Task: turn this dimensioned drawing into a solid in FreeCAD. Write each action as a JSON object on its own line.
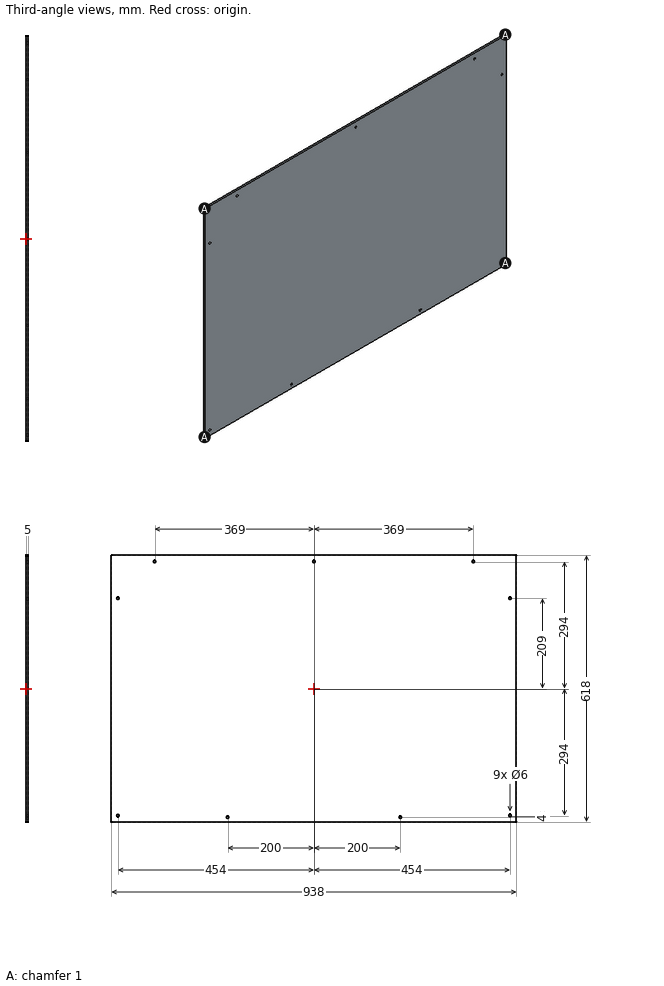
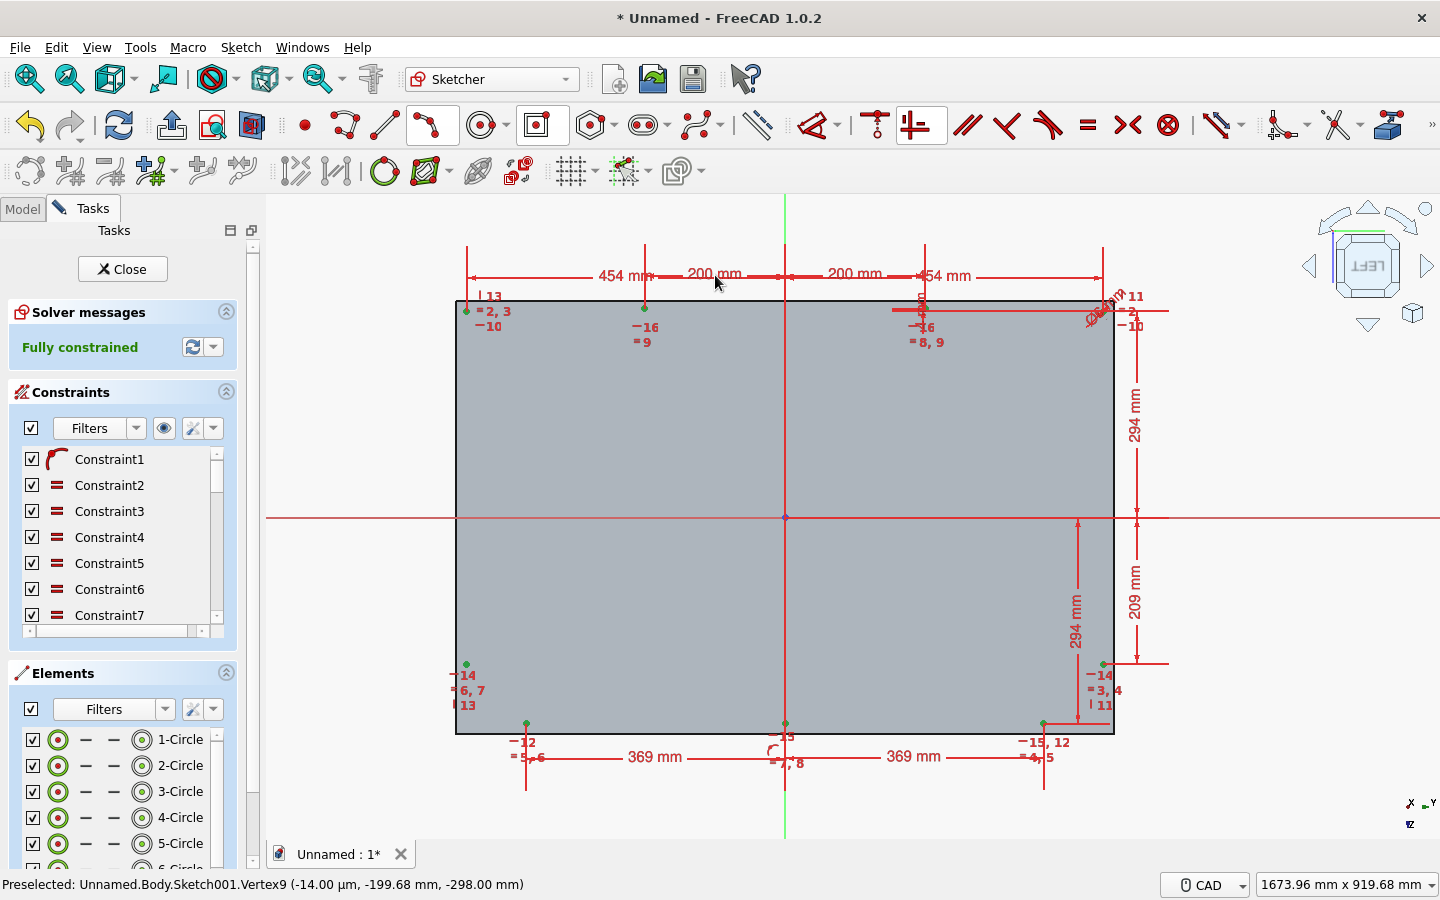
{"action": "left_click", "coordinate": [123, 269]}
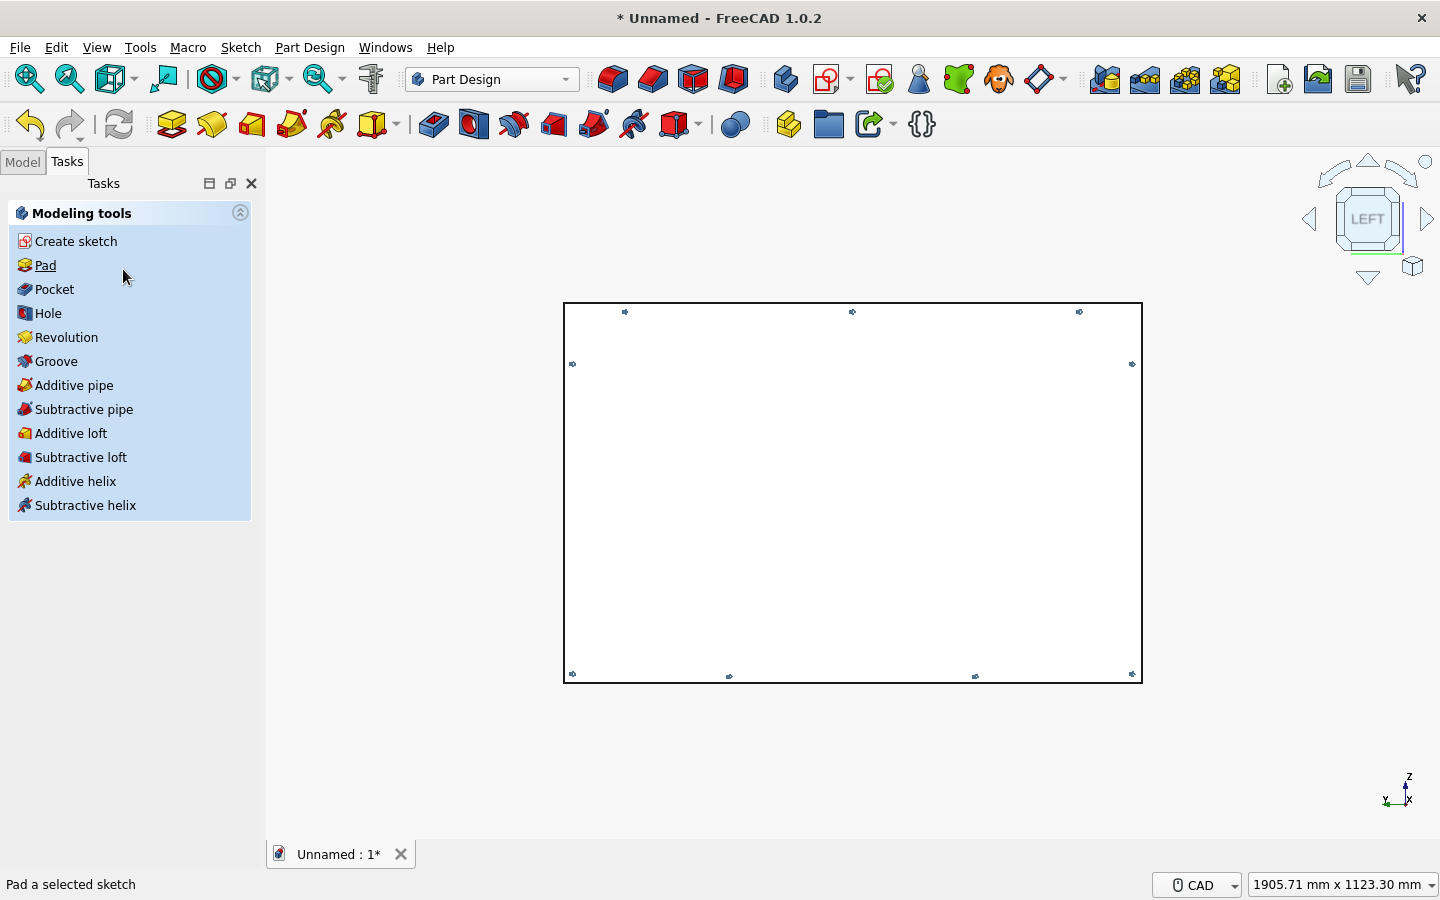
{"action": "left_click", "coordinate": [434, 124]}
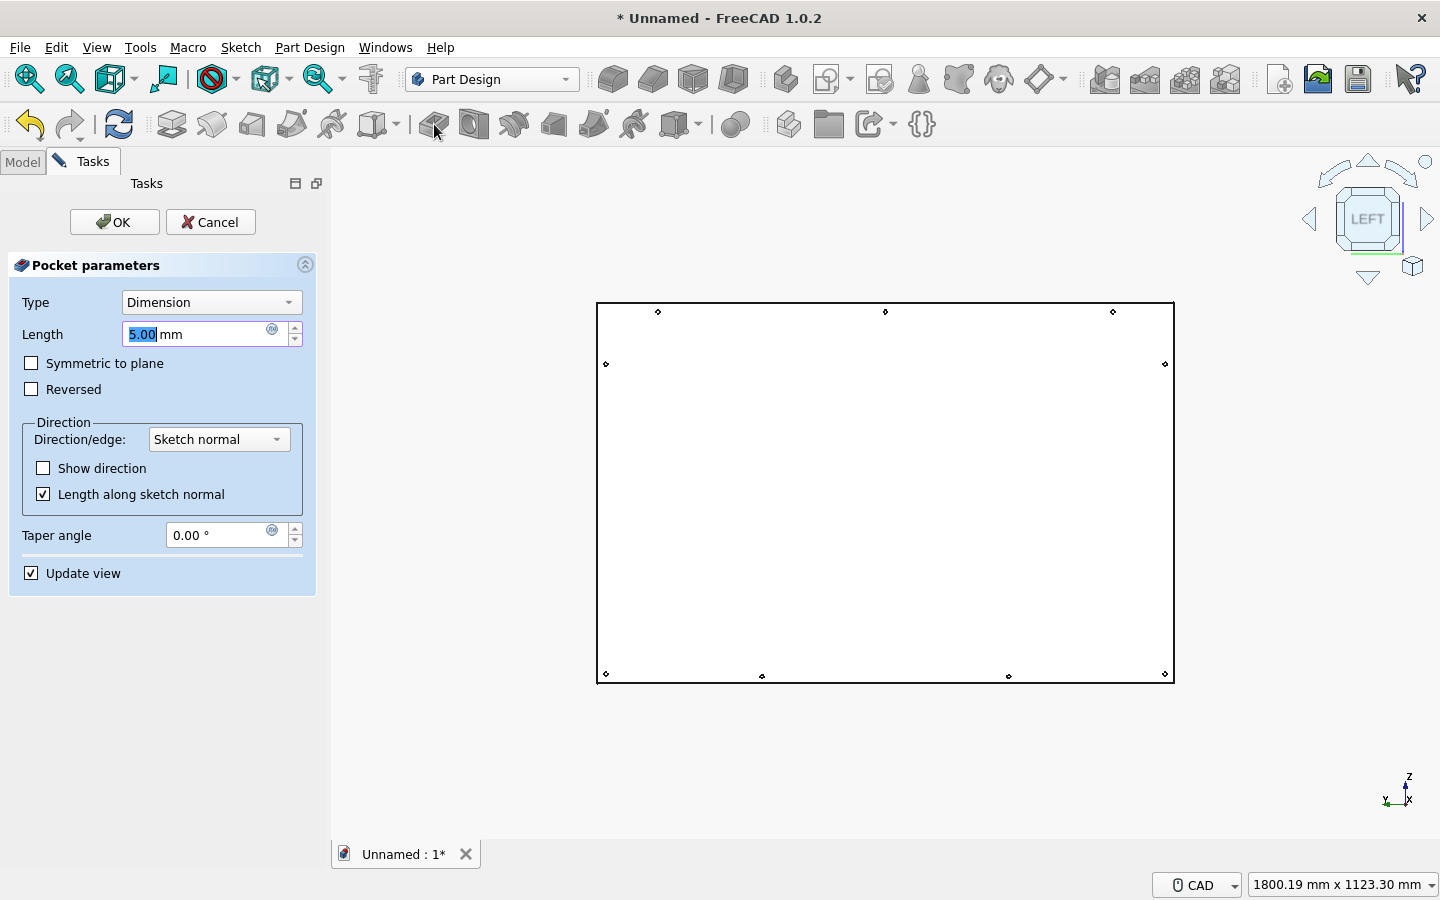
{"action": "left_click", "coordinate": [212, 302]}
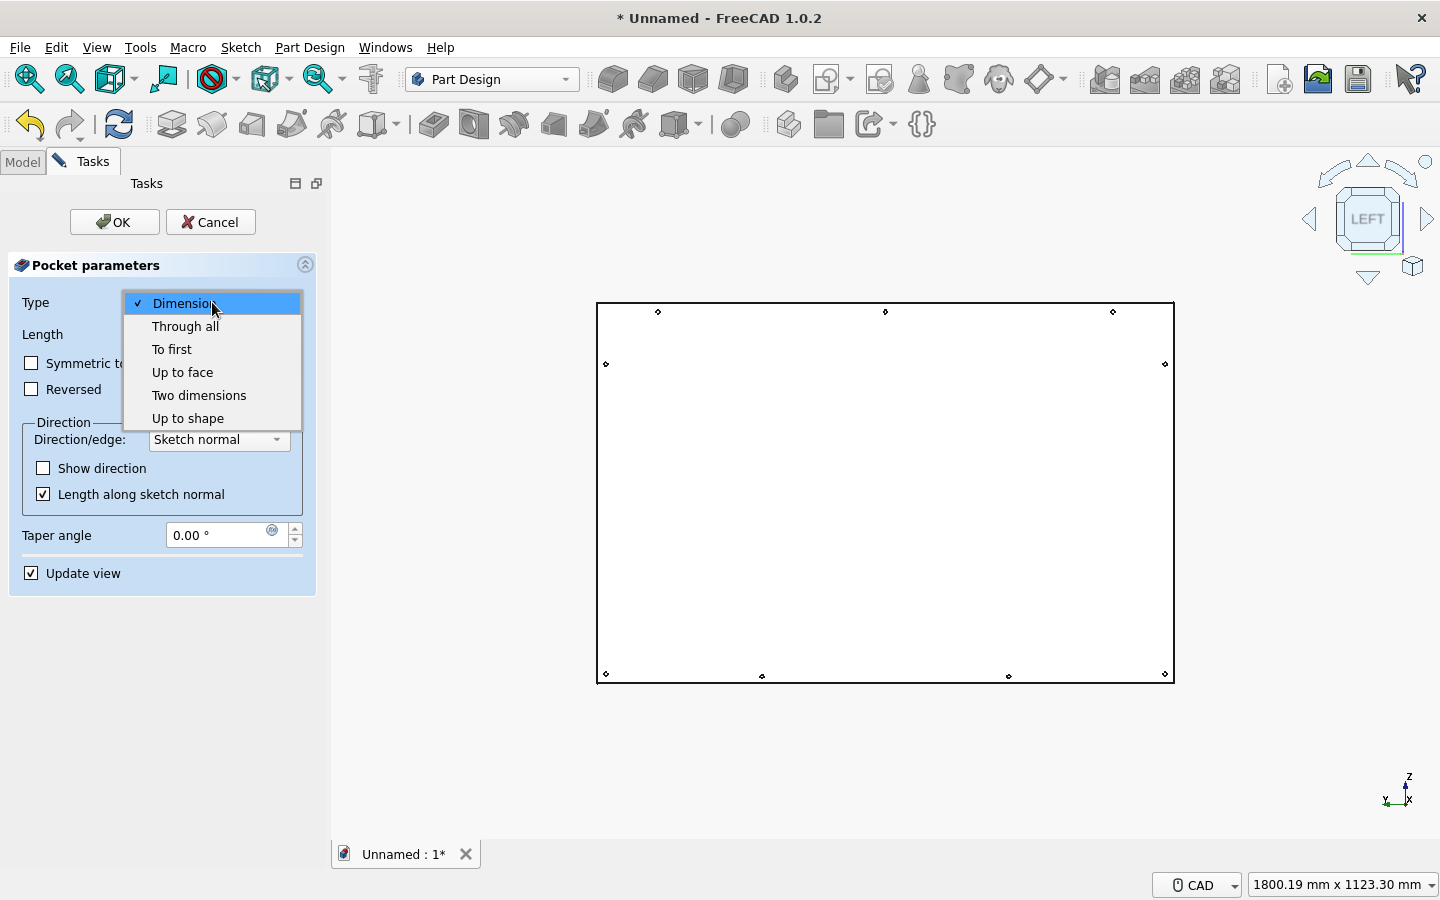
{"action": "left_click", "coordinate": [212, 326]}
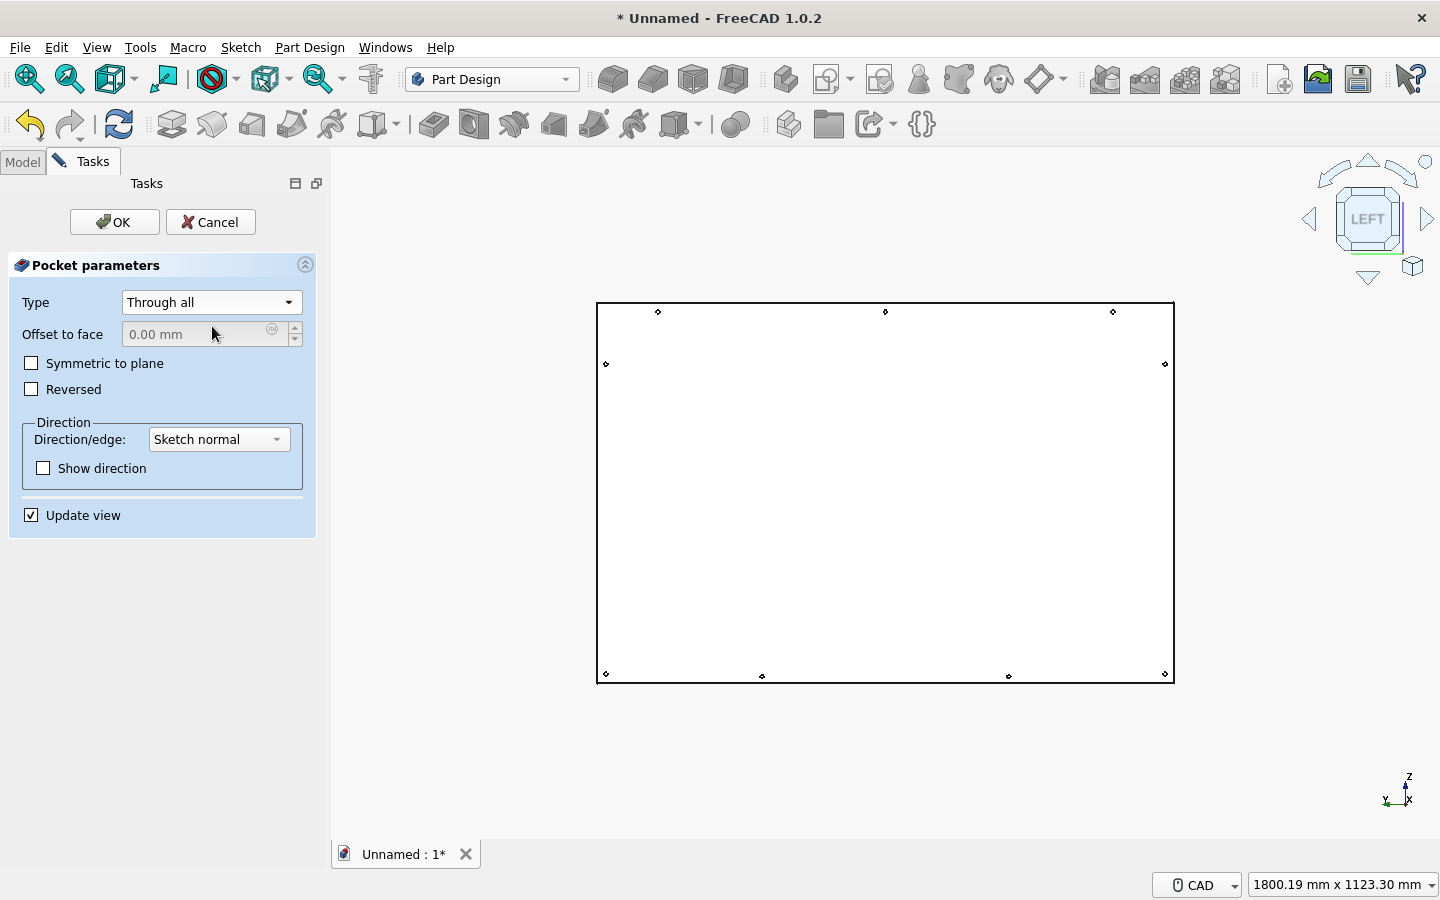
{"action": "left_click", "coordinate": [115, 222]}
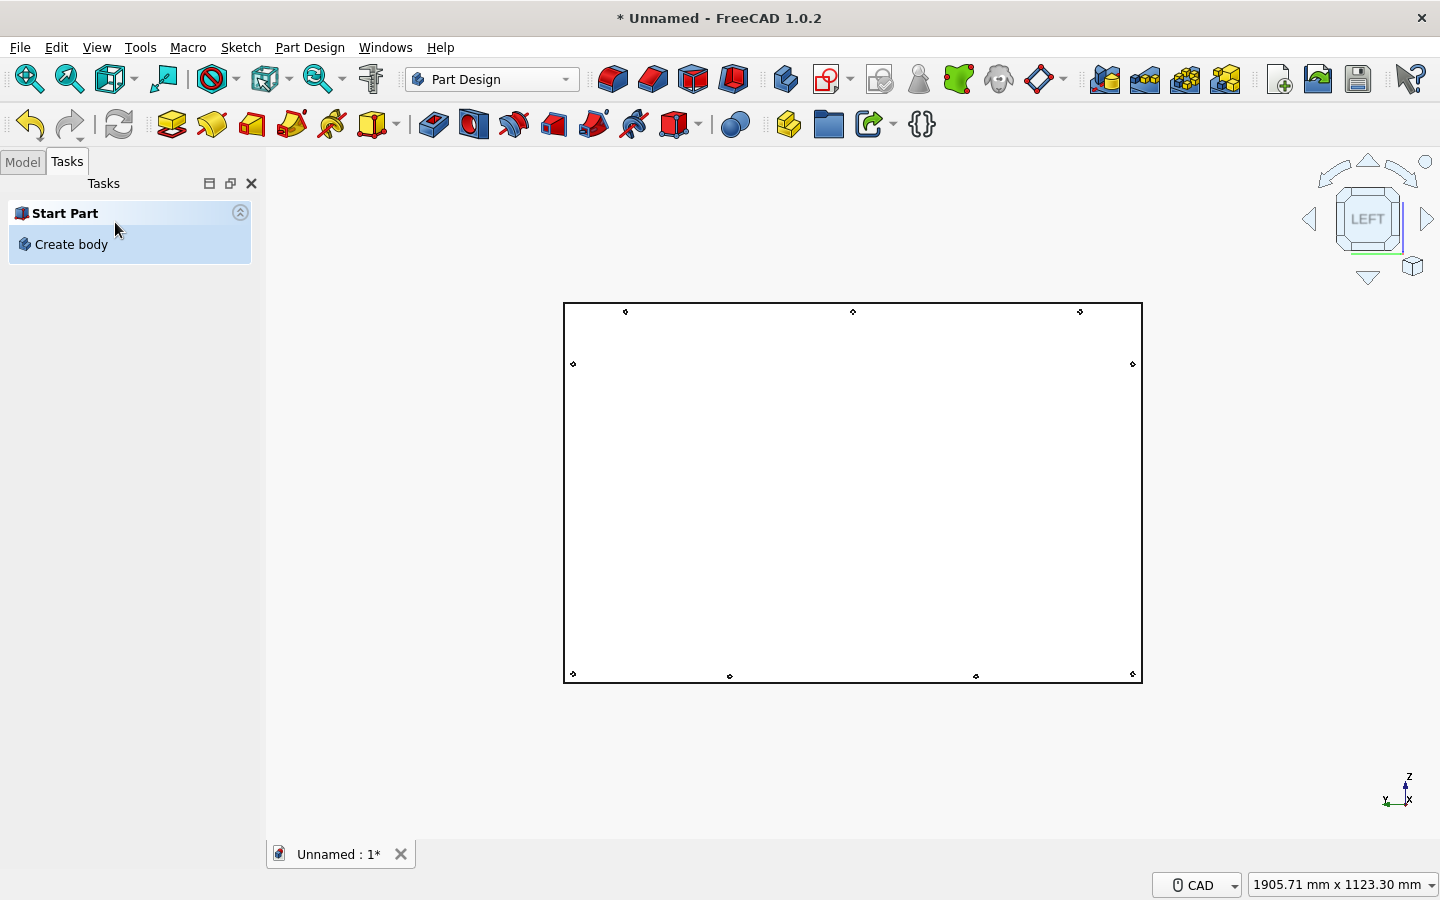
{"action": "key", "text": "0"}